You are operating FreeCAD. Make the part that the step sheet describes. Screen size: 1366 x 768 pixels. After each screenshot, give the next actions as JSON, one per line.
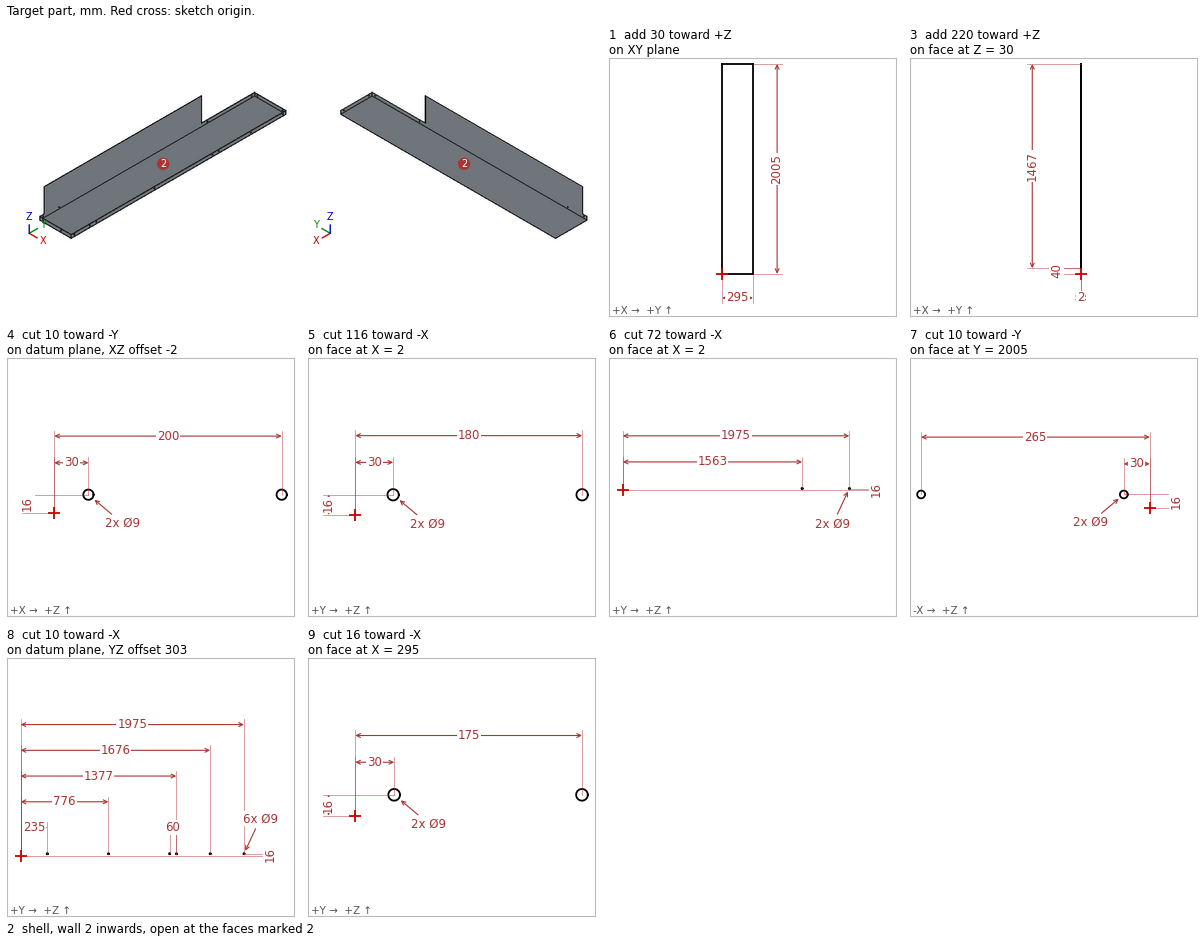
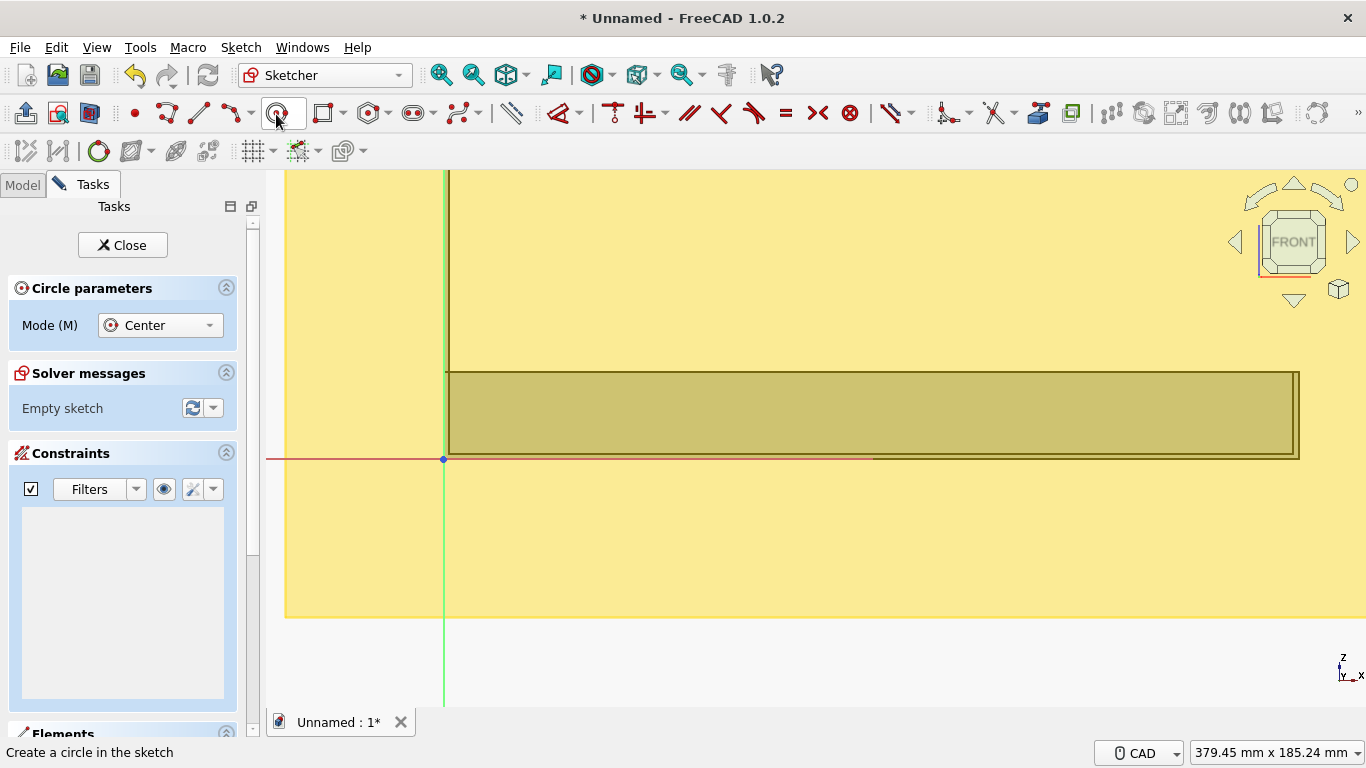
{"action": "scroll", "coordinate": [531, 413], "scroll_direction": "up", "scroll_amount": 3}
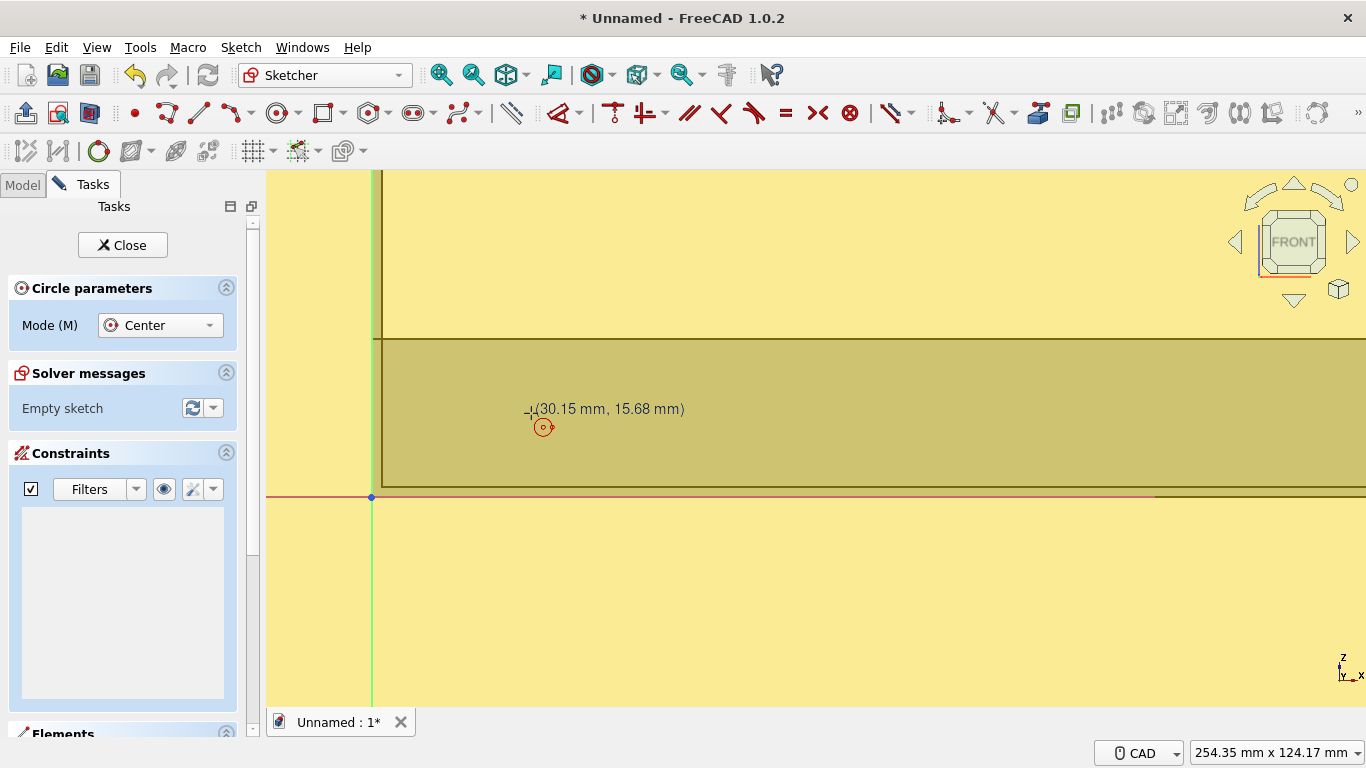
{"action": "left_click", "coordinate": [530, 413]}
{"action": "left_click", "coordinate": [547, 396]}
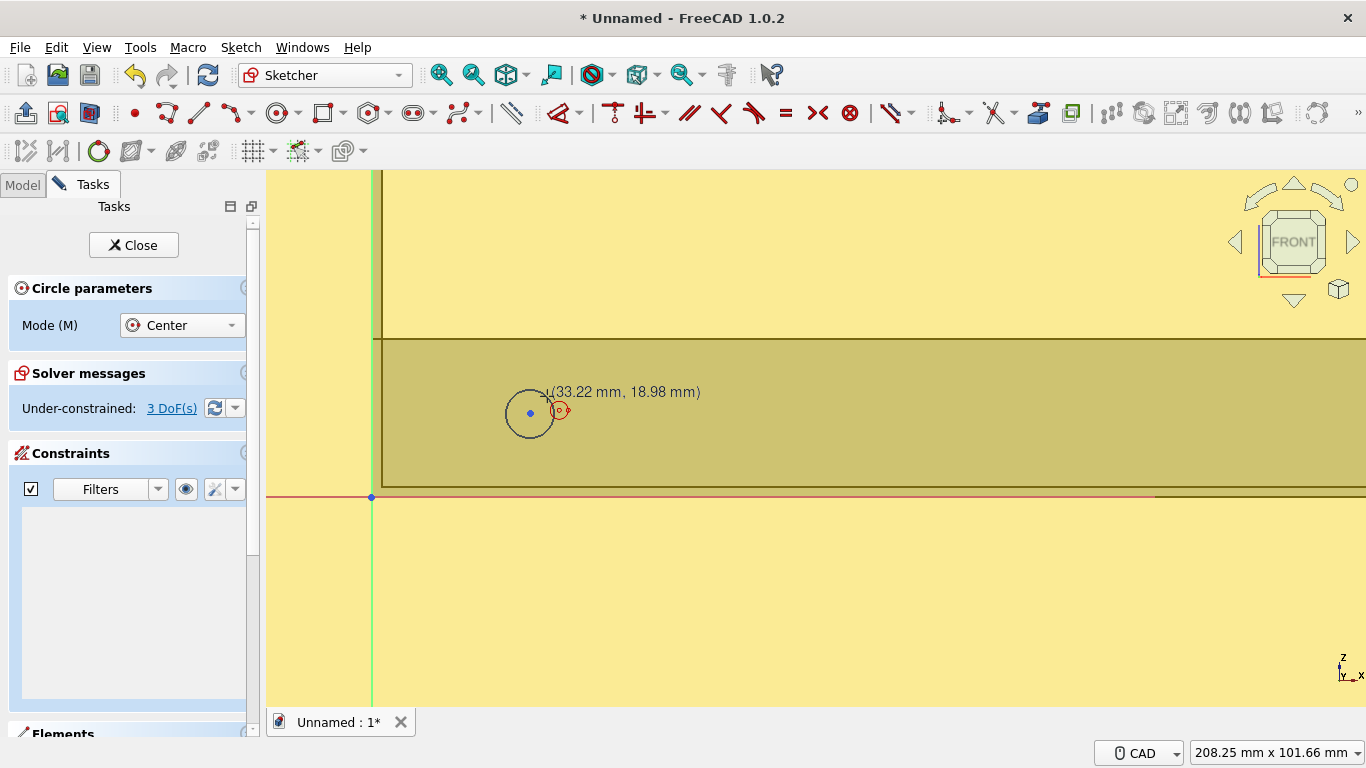
{"action": "scroll", "coordinate": [548, 433], "scroll_direction": "down", "scroll_amount": 3}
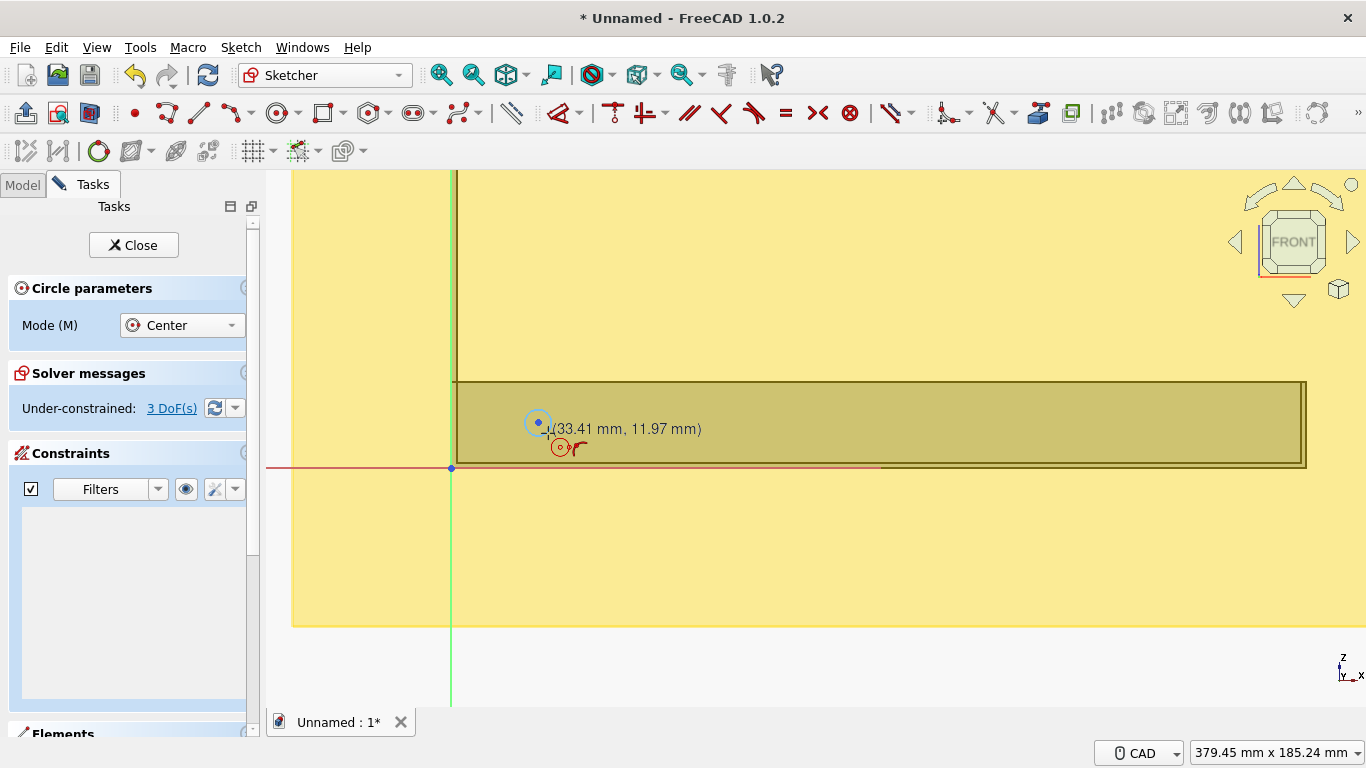
{"action": "scroll", "coordinate": [1031, 422], "scroll_direction": "up", "scroll_amount": 3}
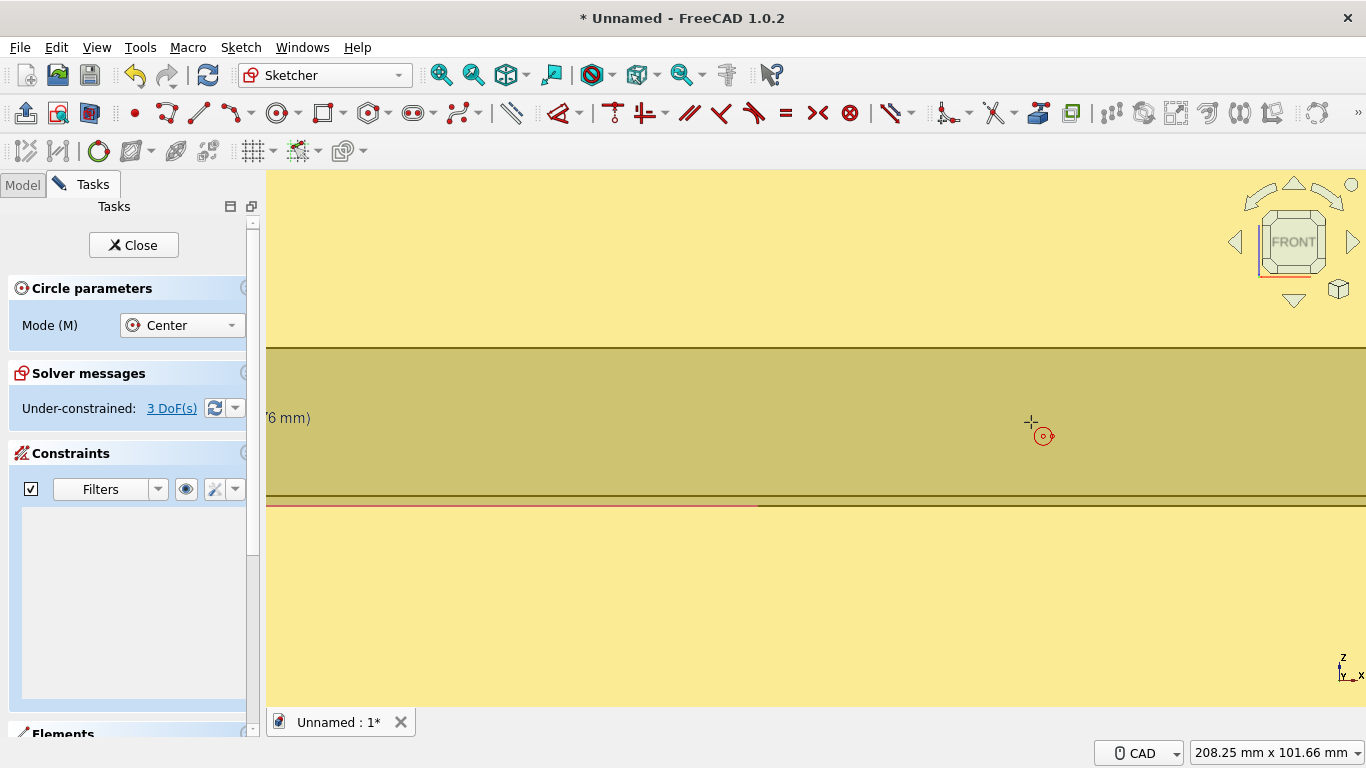
{"action": "left_click", "coordinate": [1031, 422]}
{"action": "left_click", "coordinate": [1047, 405]}
{"action": "key", "text": "Escape"}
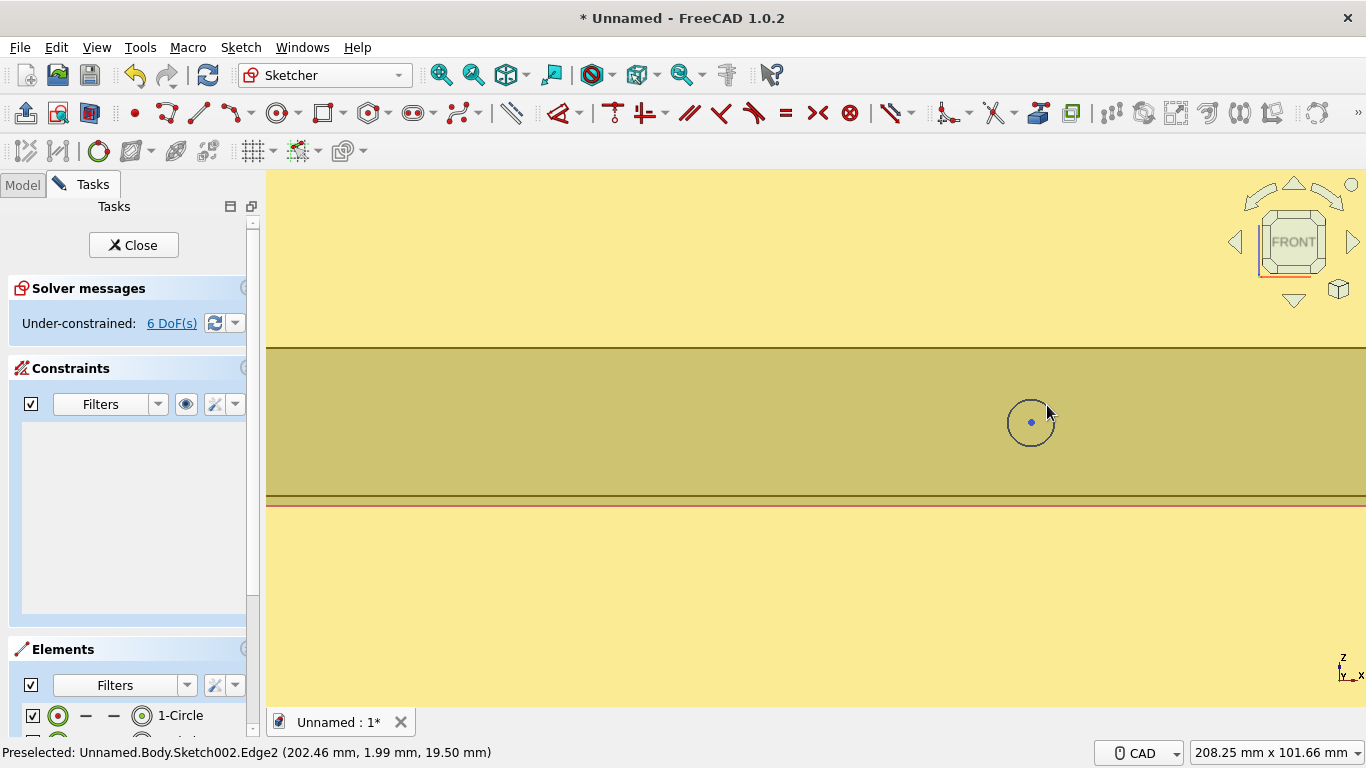
{"action": "scroll", "coordinate": [1031, 422], "scroll_direction": "down", "scroll_amount": 3}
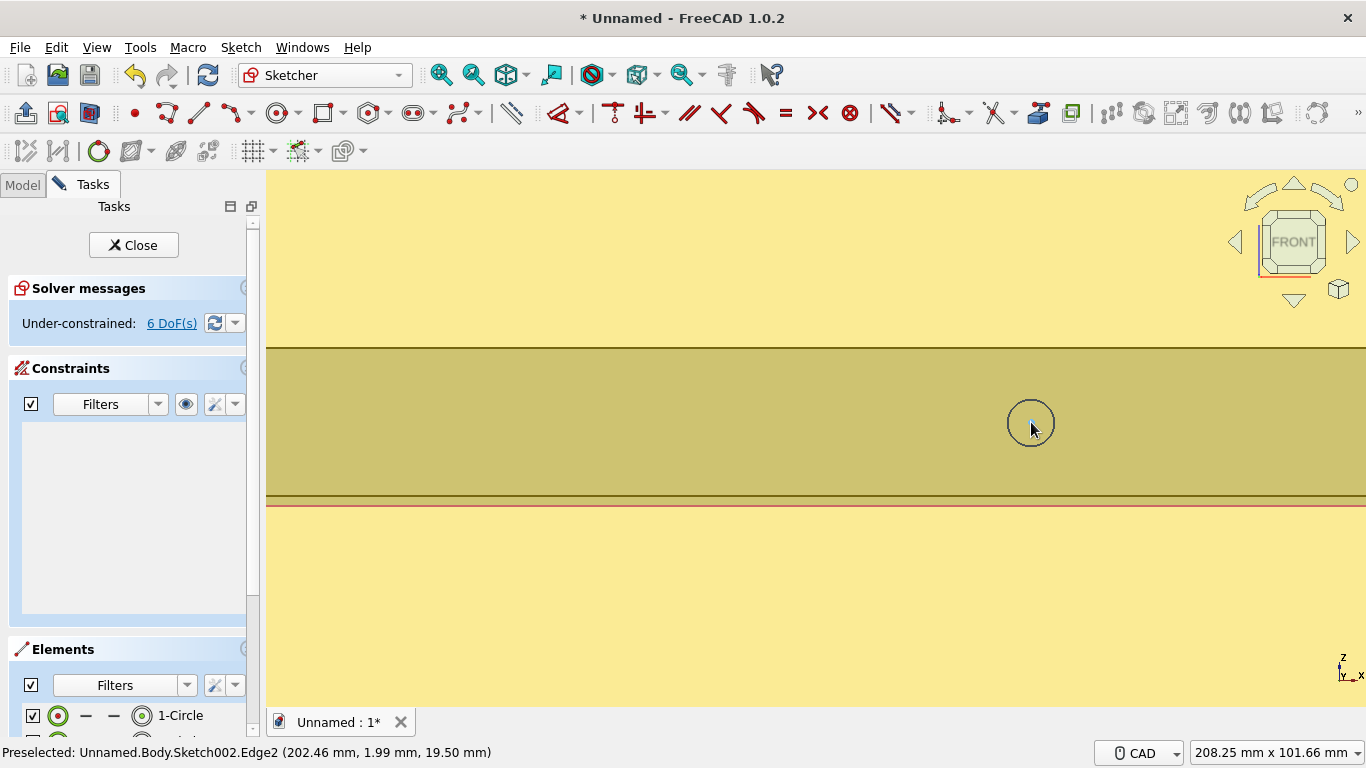
{"action": "left_click", "coordinate": [548, 413]}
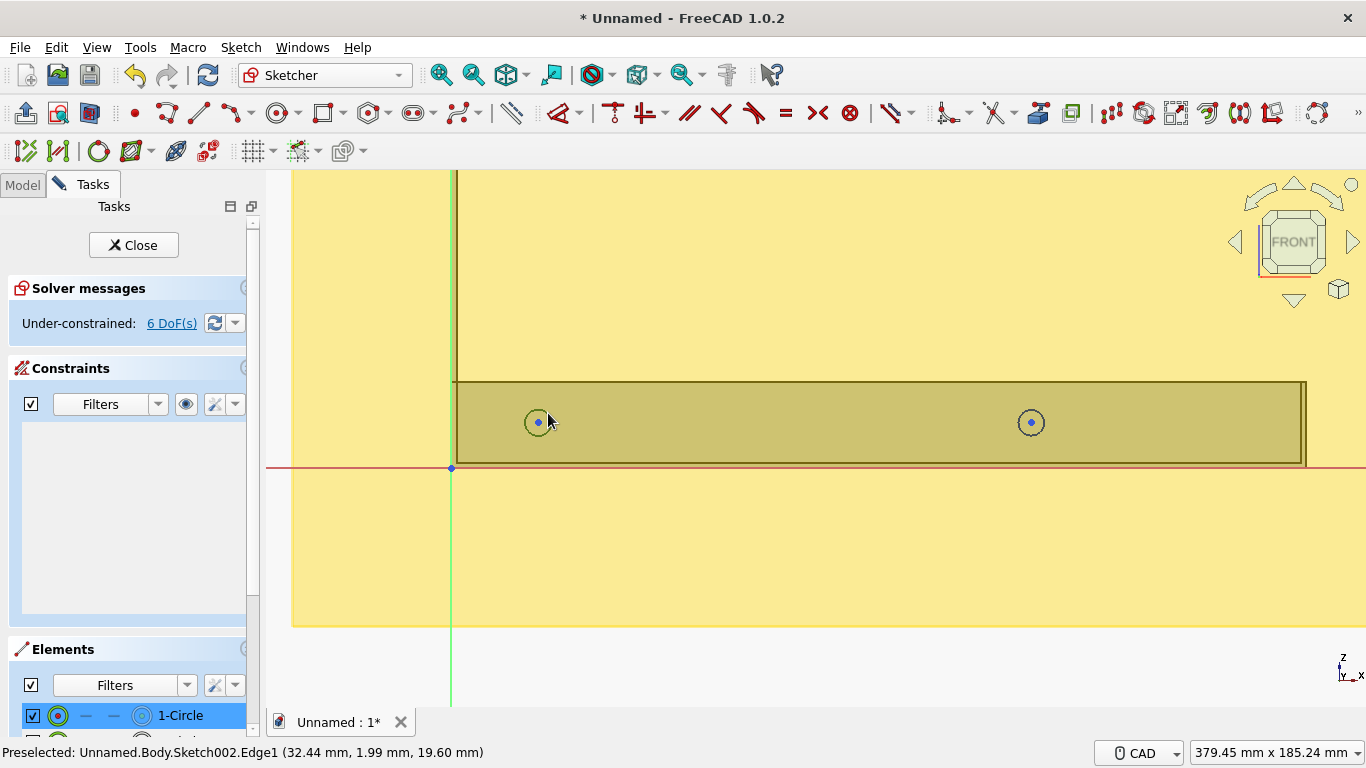
{"action": "left_click", "coordinate": [1040, 414]}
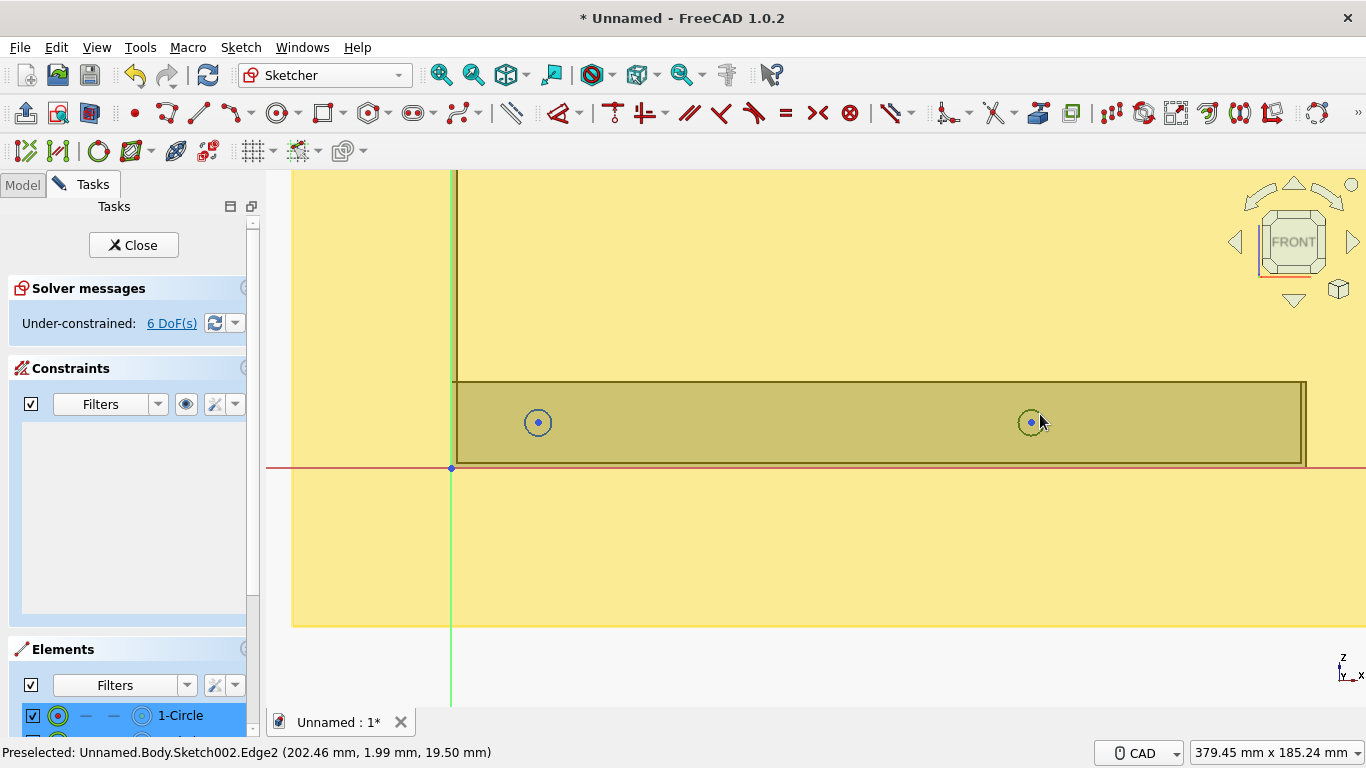
{"action": "left_click", "coordinate": [786, 114]}